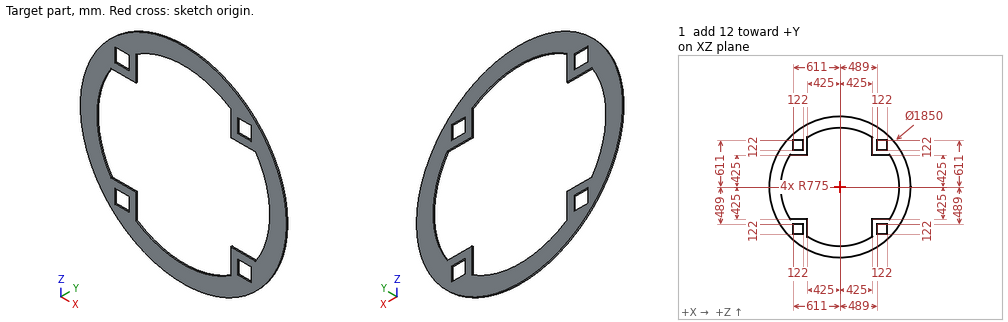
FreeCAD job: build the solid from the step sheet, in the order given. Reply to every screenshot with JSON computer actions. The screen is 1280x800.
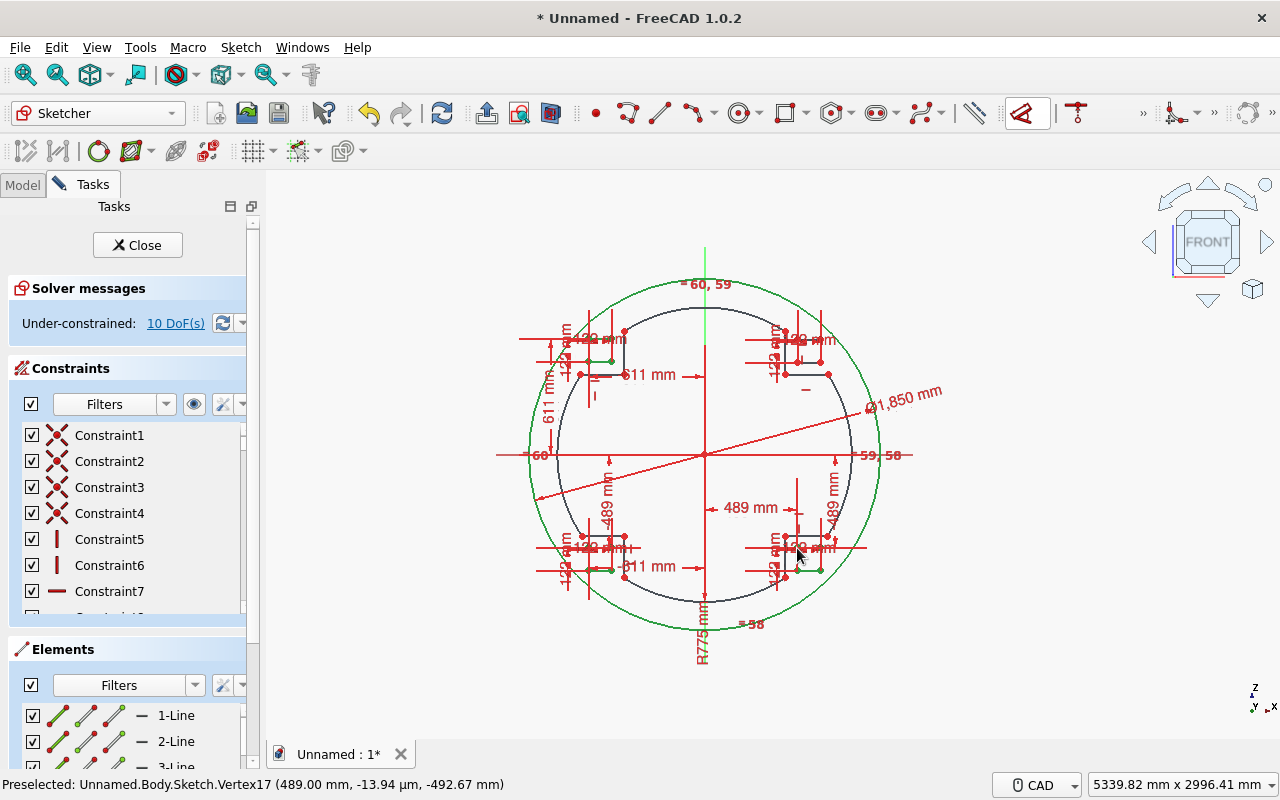
{"action": "left_click", "coordinate": [582, 536]}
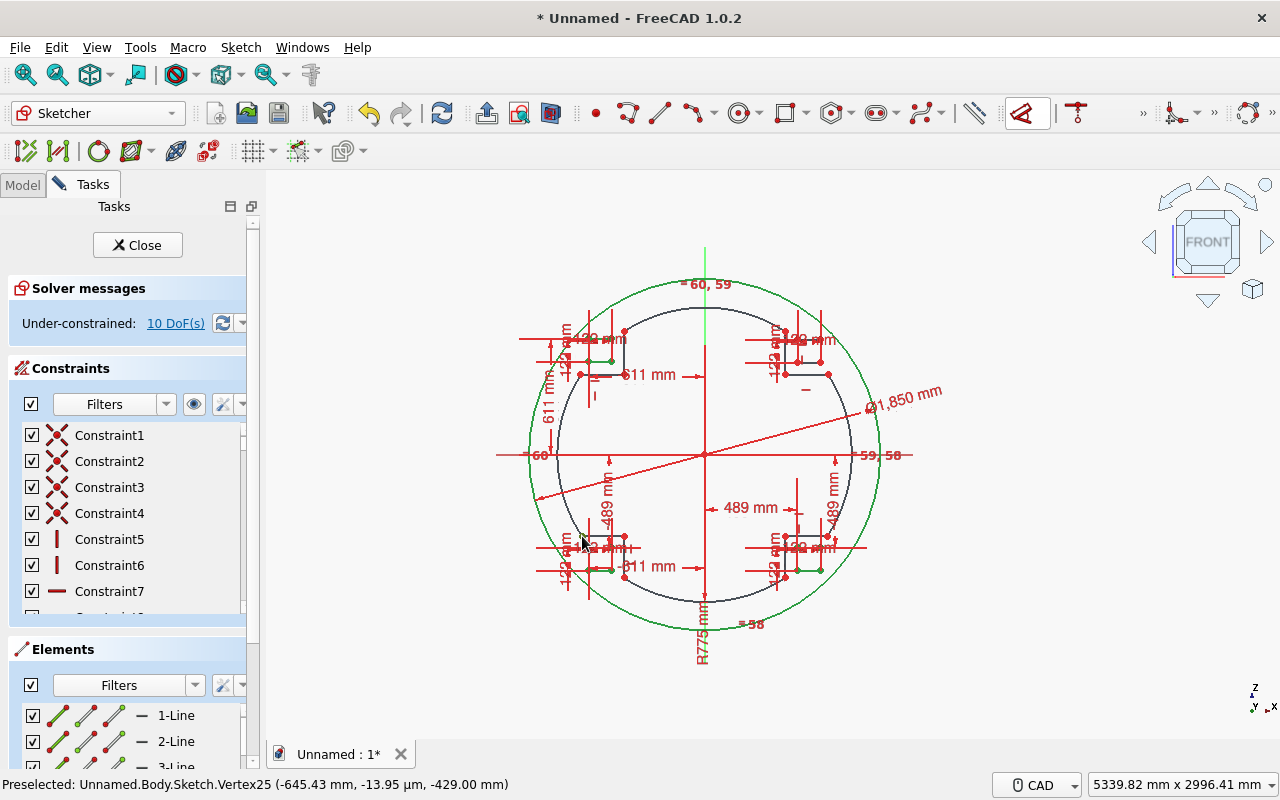
{"action": "key", "text": "i"}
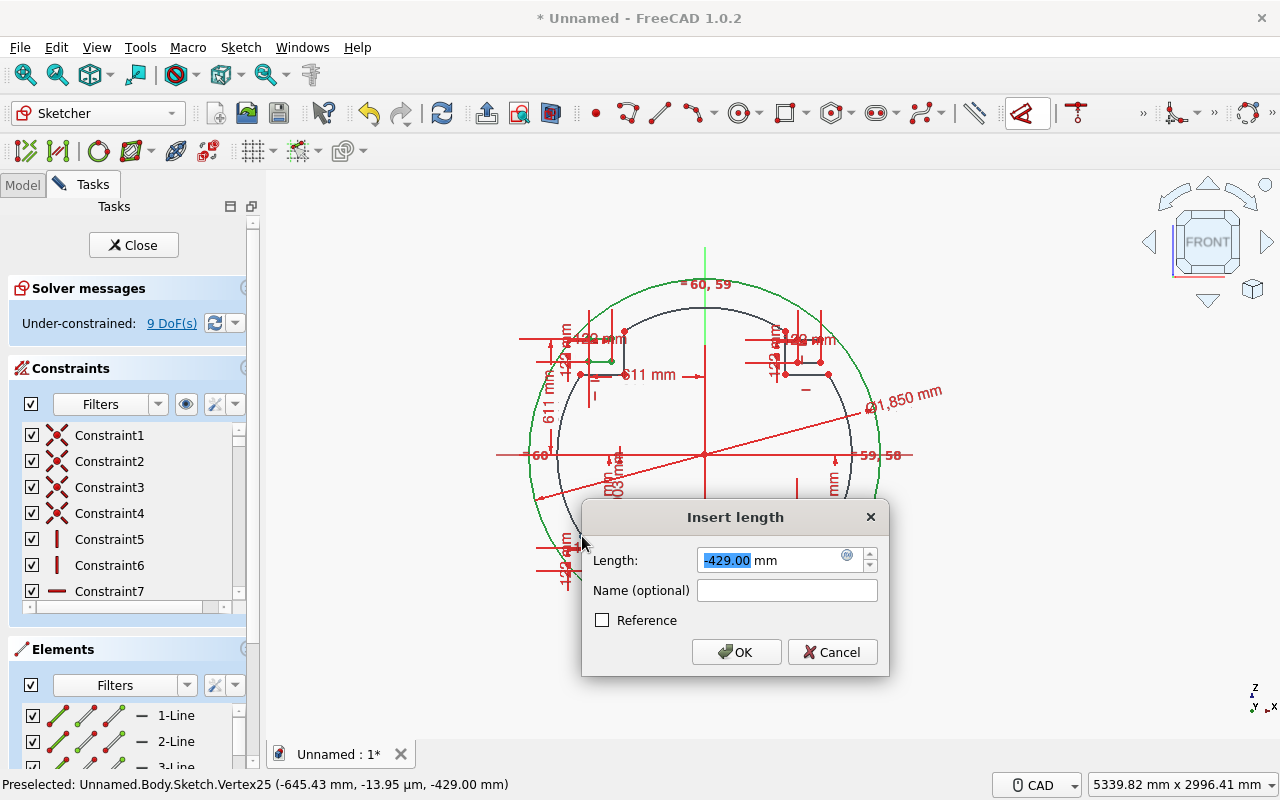
{"action": "type", "text": "-425"}
{"action": "key", "text": "Return"}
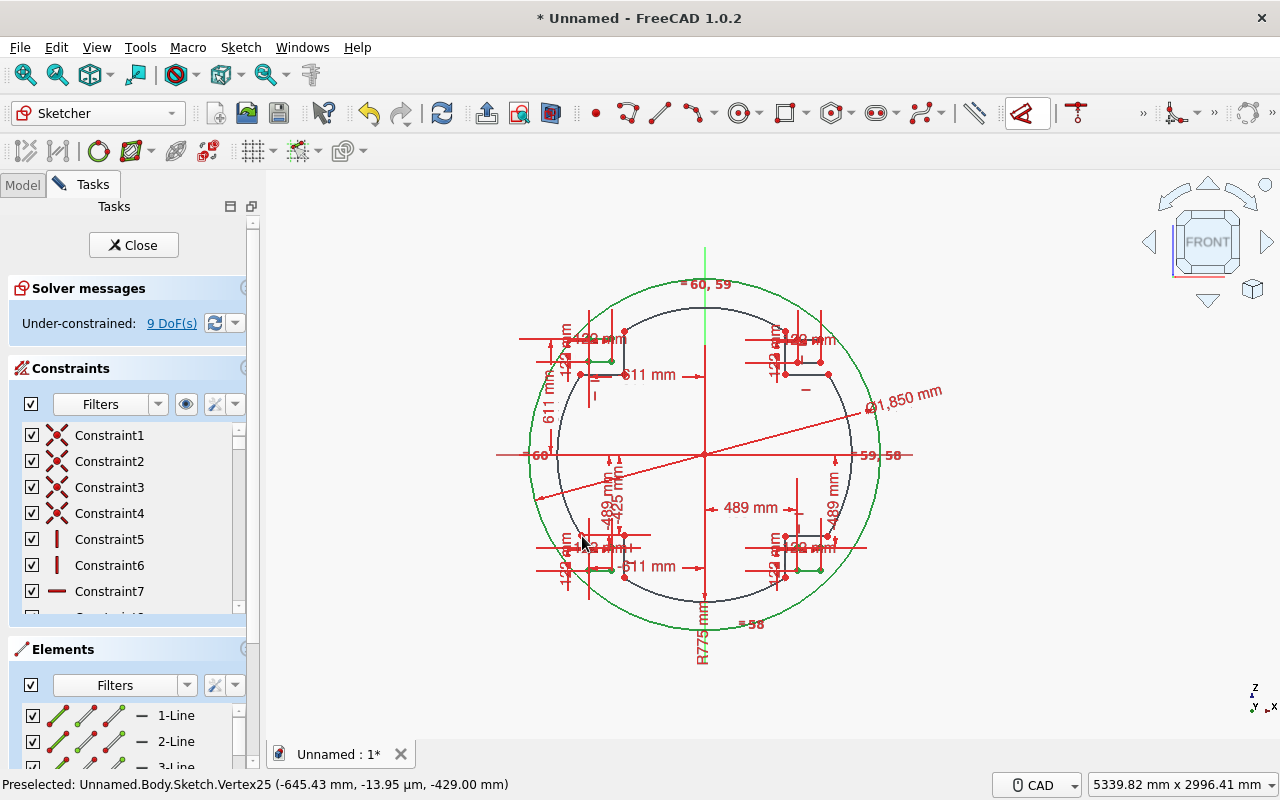
{"action": "left_click", "coordinate": [624, 535]}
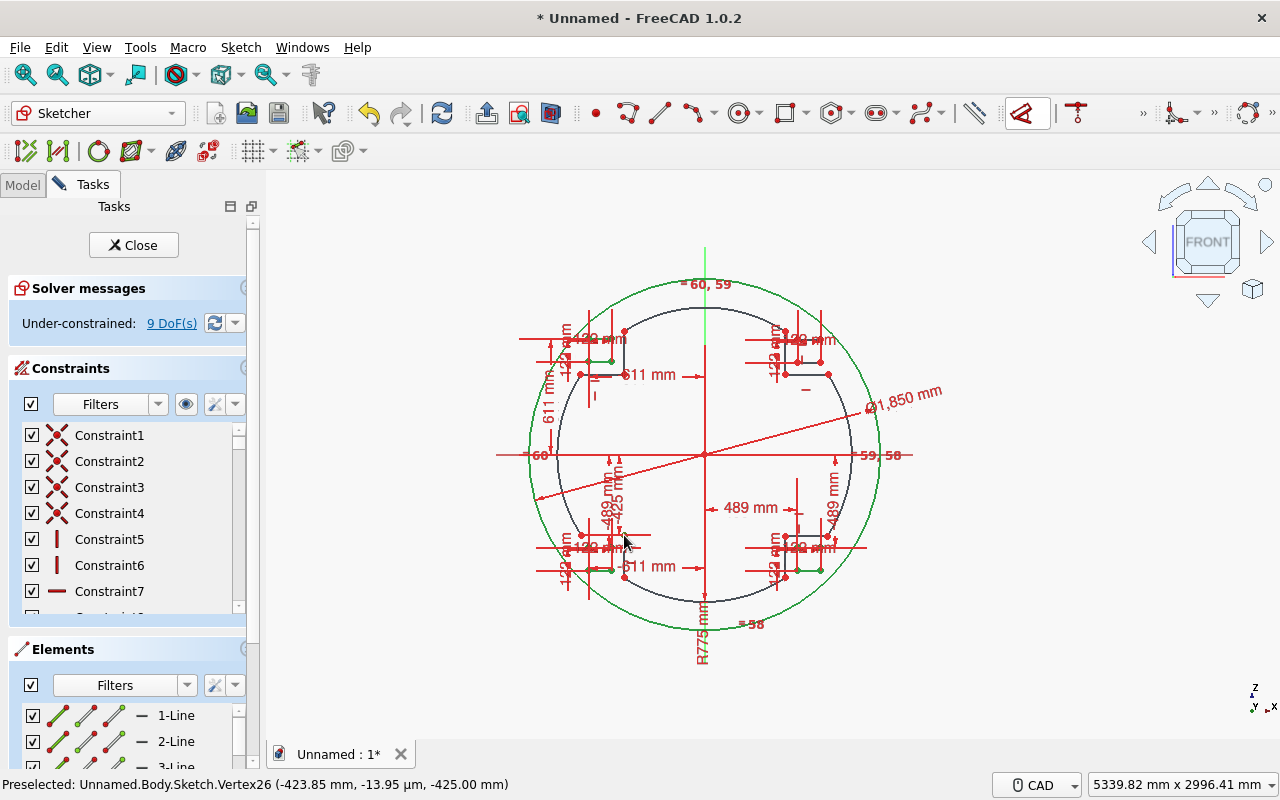
{"action": "left_click", "coordinate": [1044, 114]}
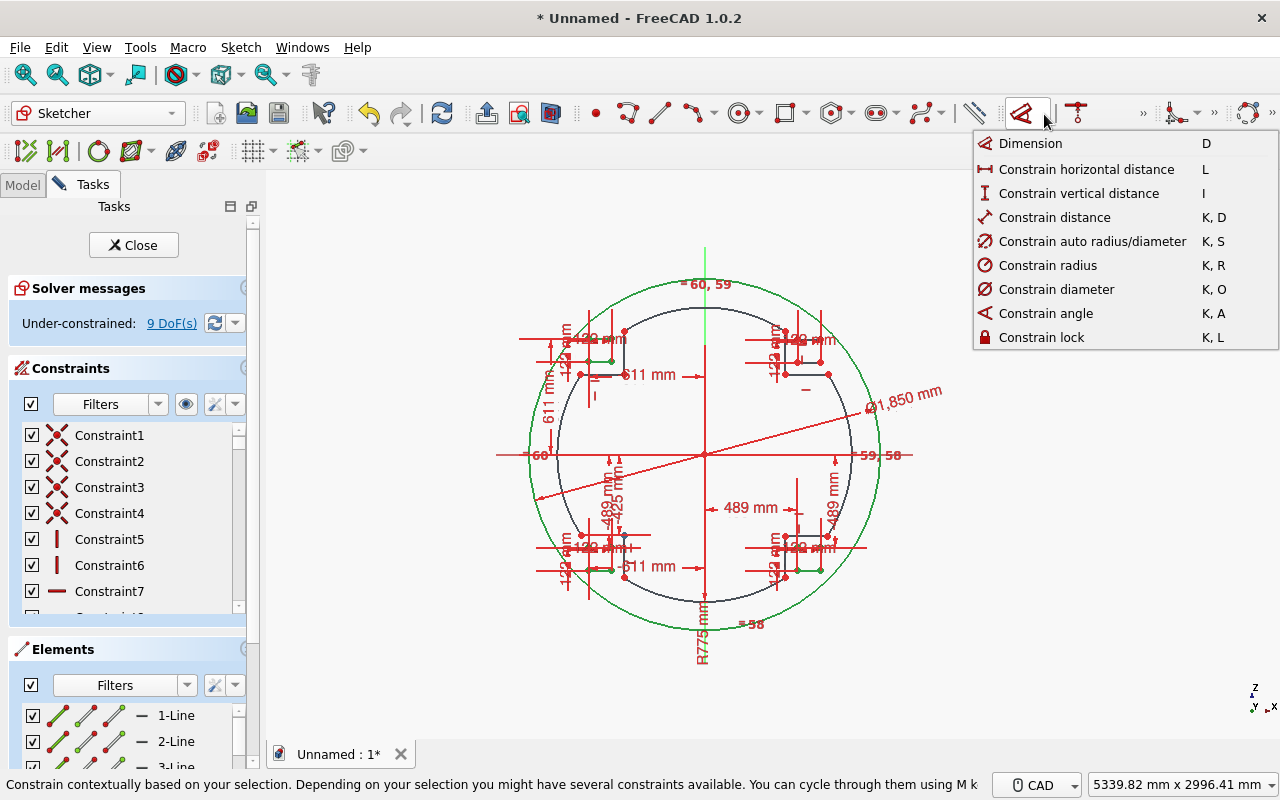
{"action": "left_click", "coordinate": [1126, 169]}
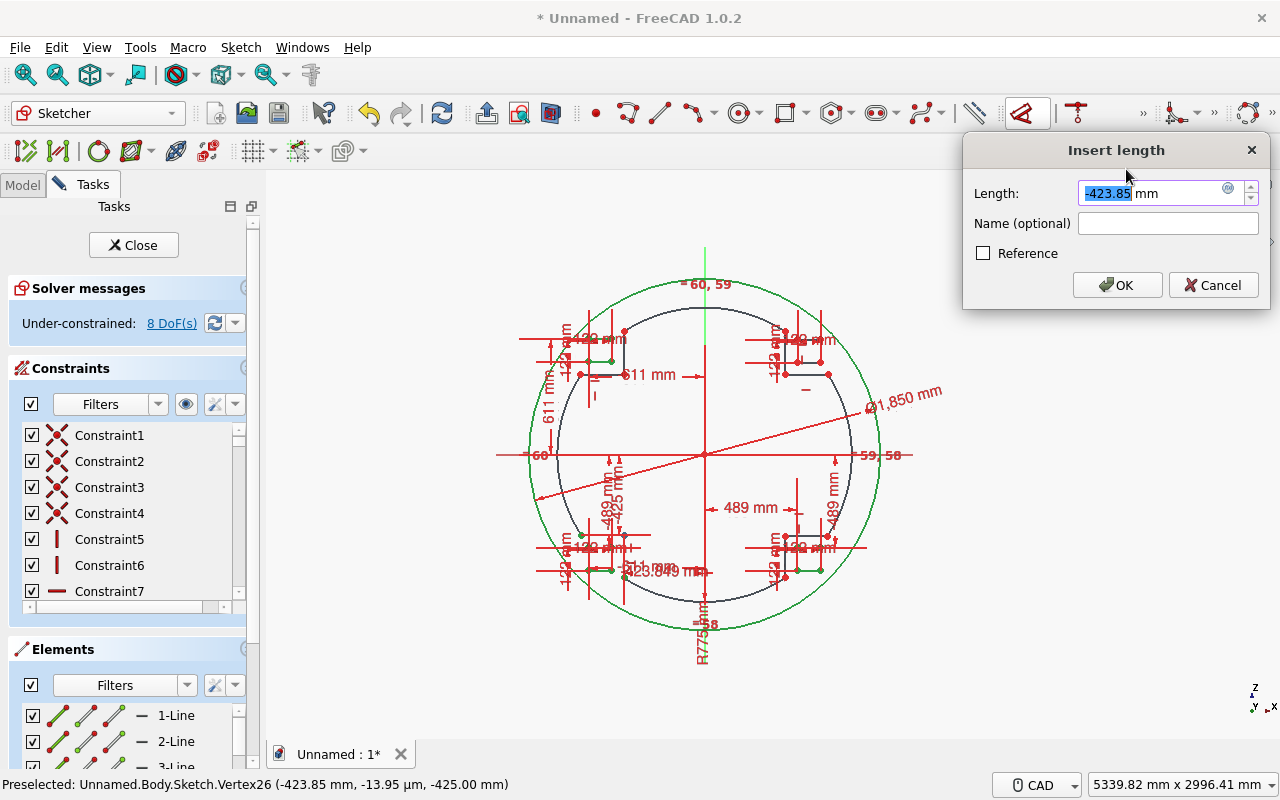
{"action": "type", "text": "-425"}
{"action": "key", "text": "Return"}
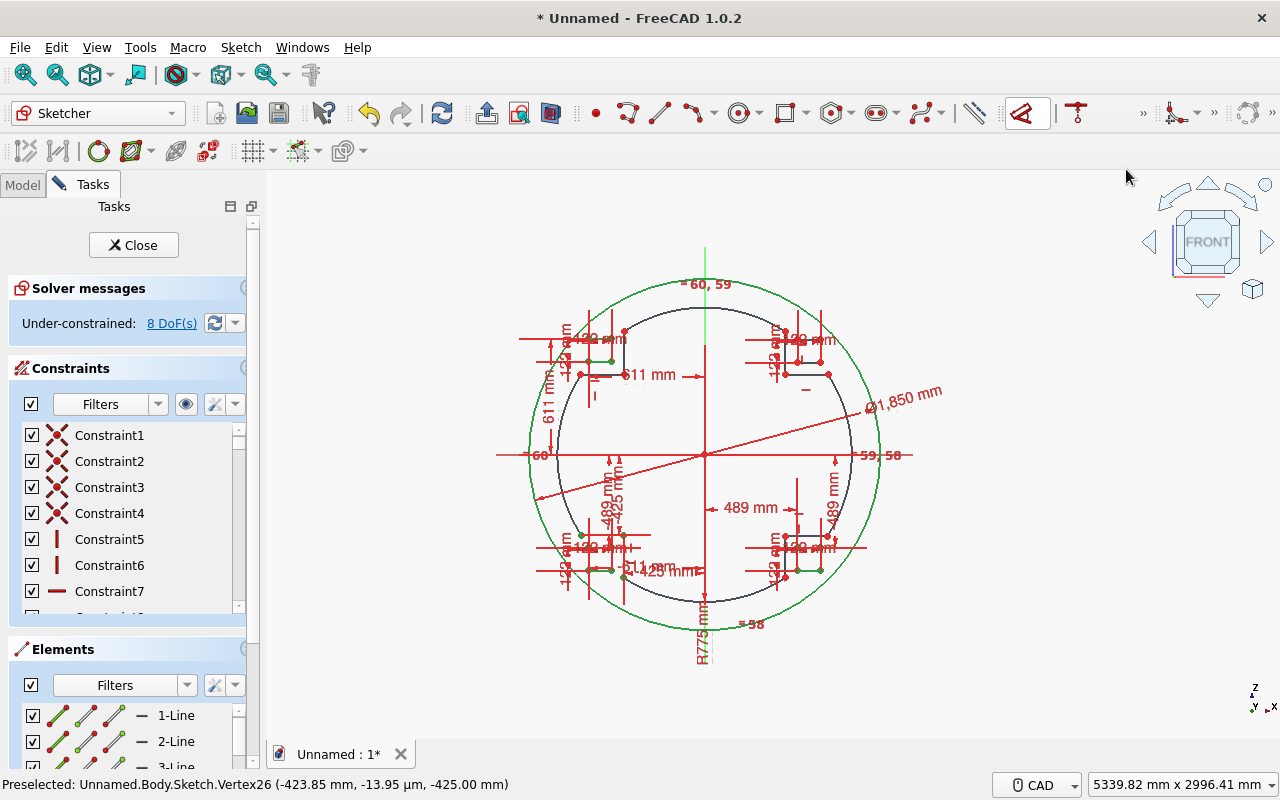
{"action": "left_click", "coordinate": [785, 578]}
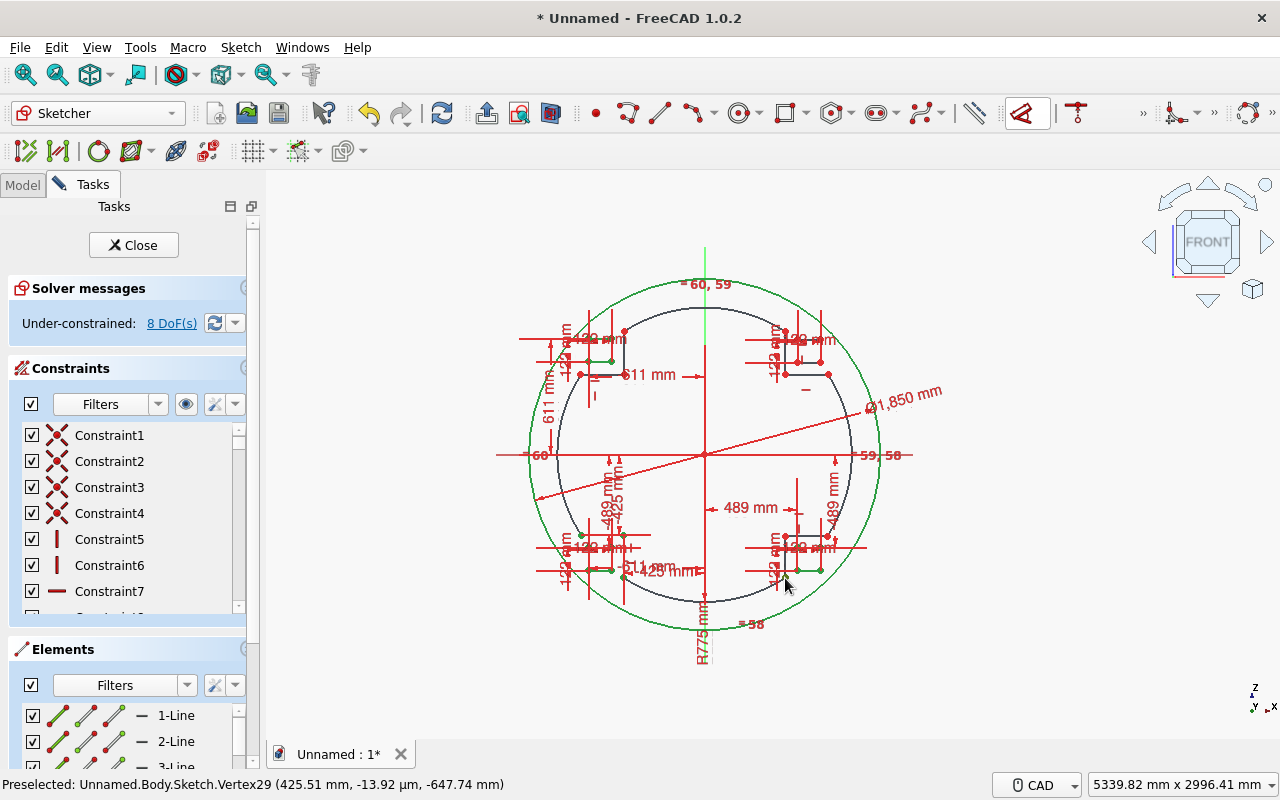
{"action": "key", "text": "l"}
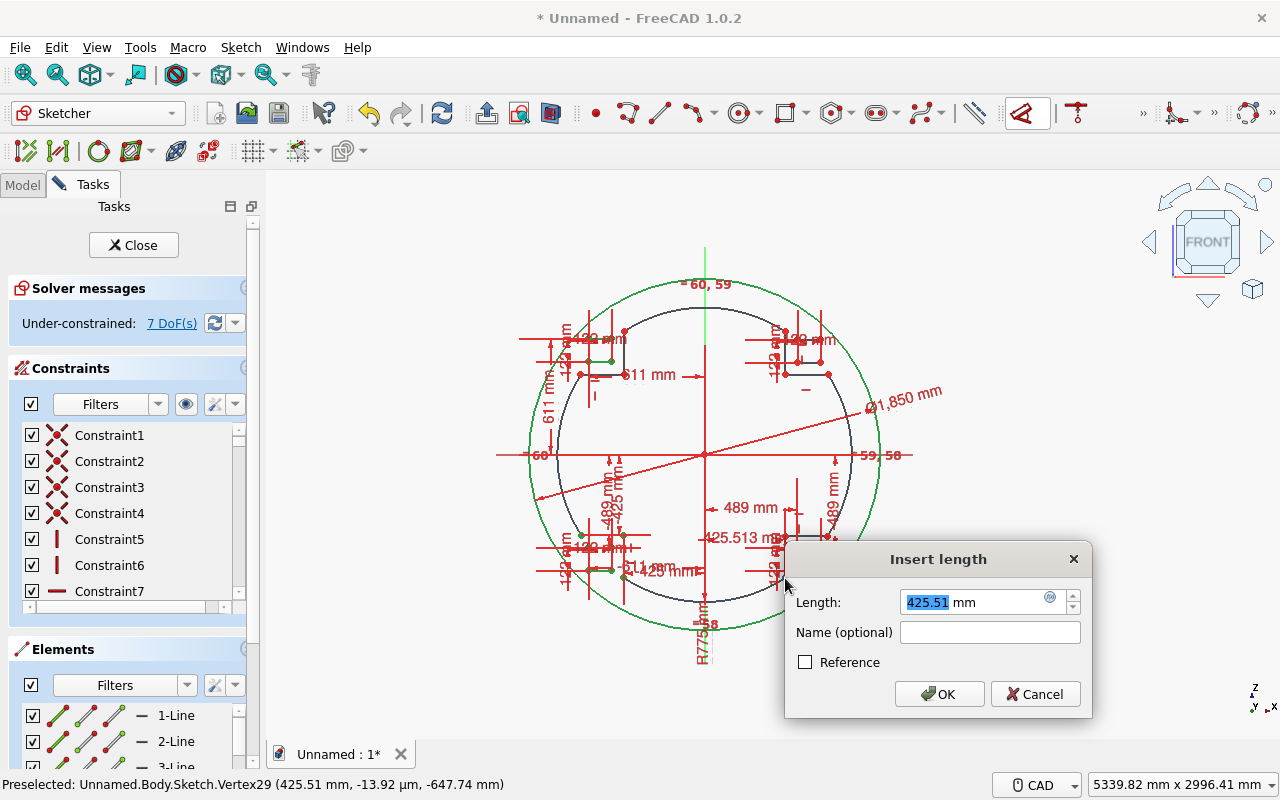
{"action": "type", "text": "425"}
{"action": "key", "text": "Return"}